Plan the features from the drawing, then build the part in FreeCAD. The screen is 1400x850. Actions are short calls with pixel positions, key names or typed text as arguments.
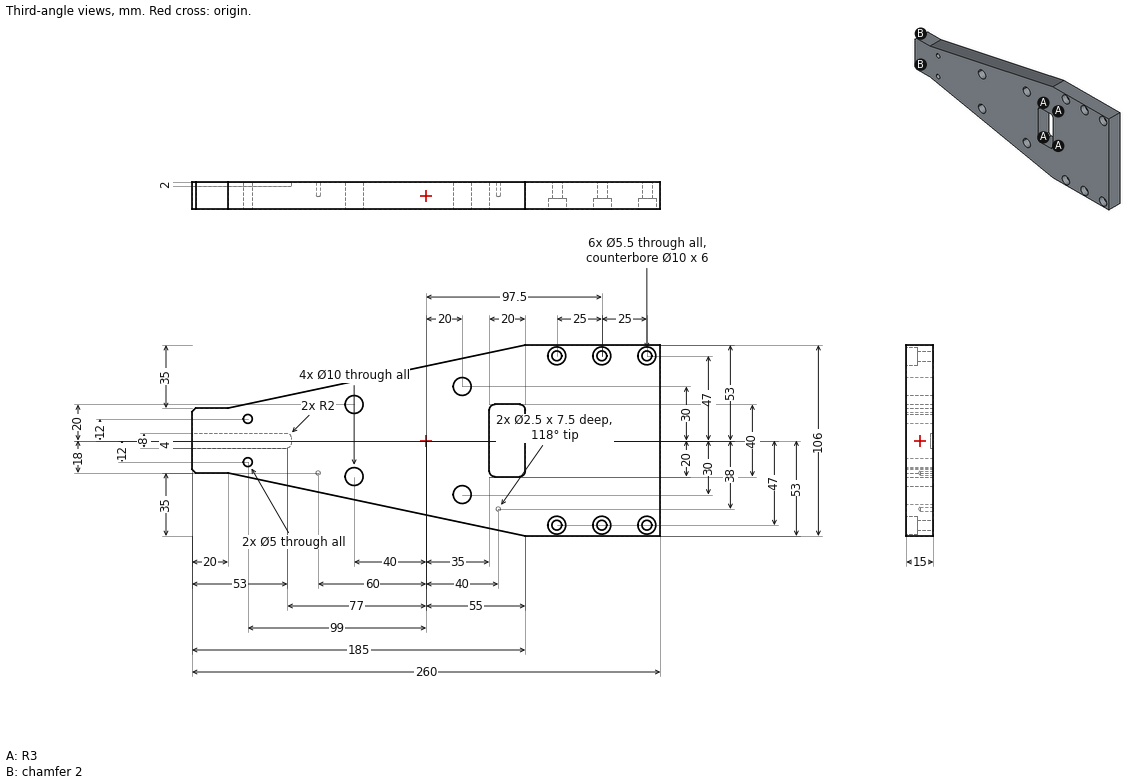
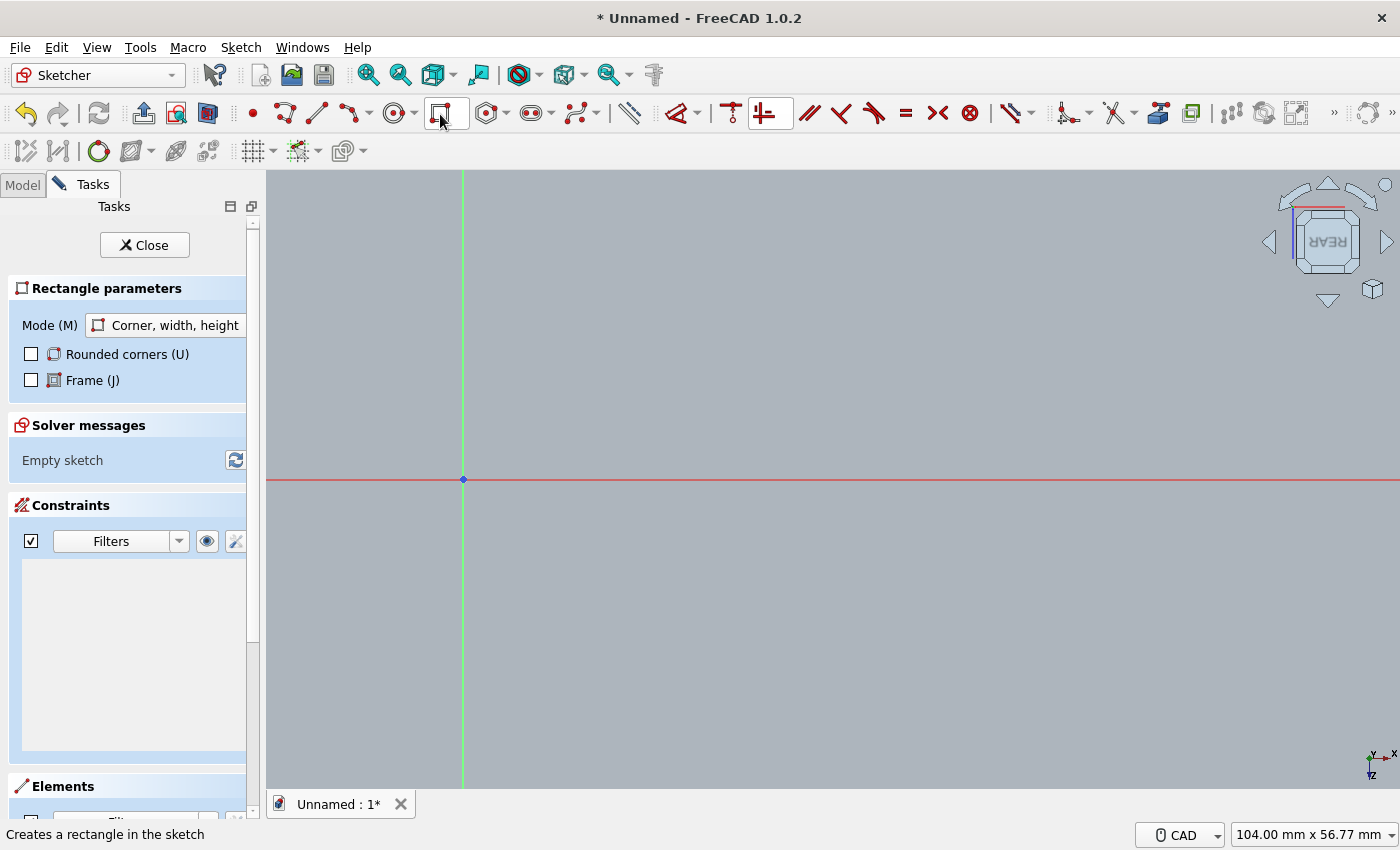
click(845, 261)
click(1063, 698)
key(Escape)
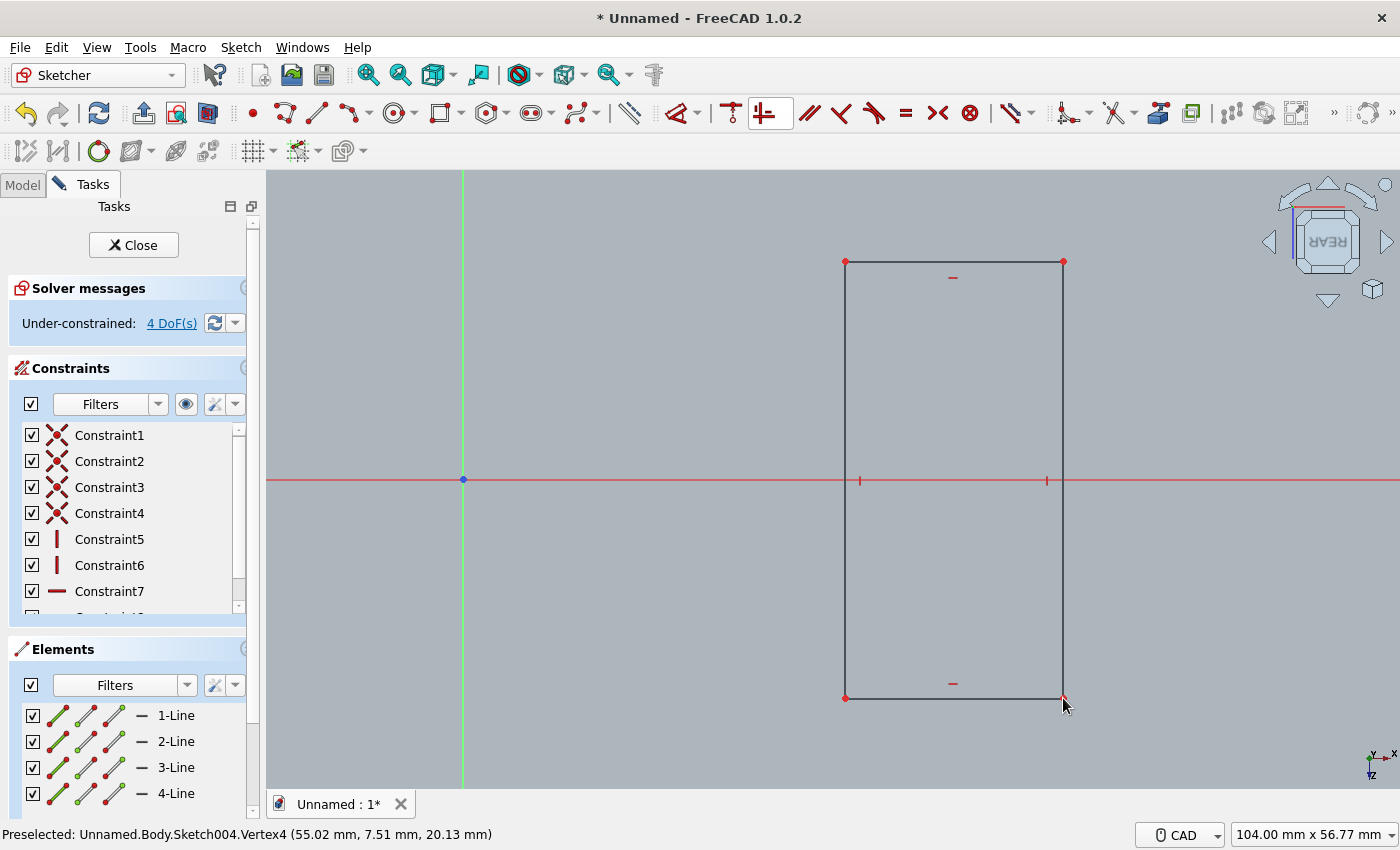
click(676, 114)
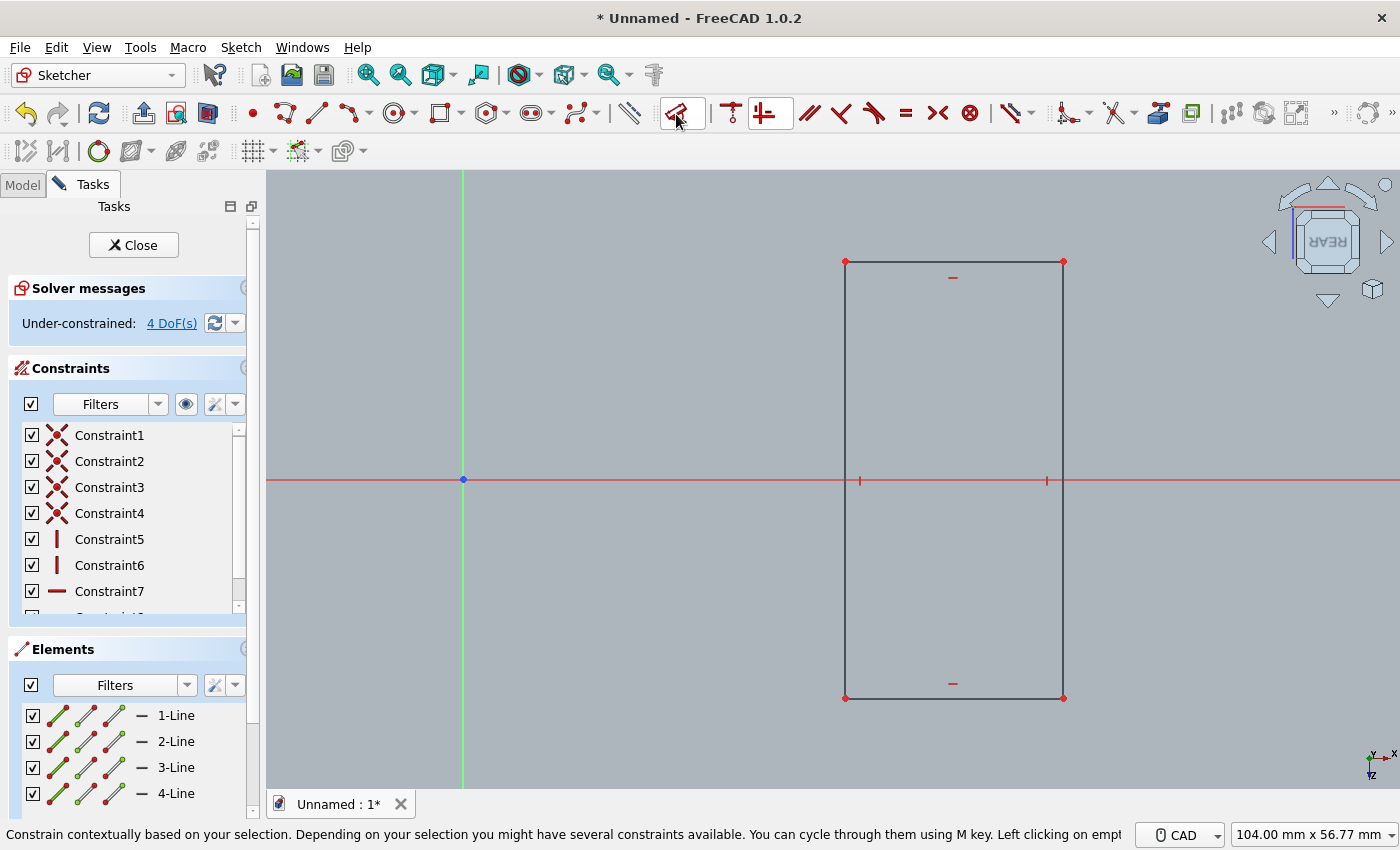
click(845, 393)
click(879, 380)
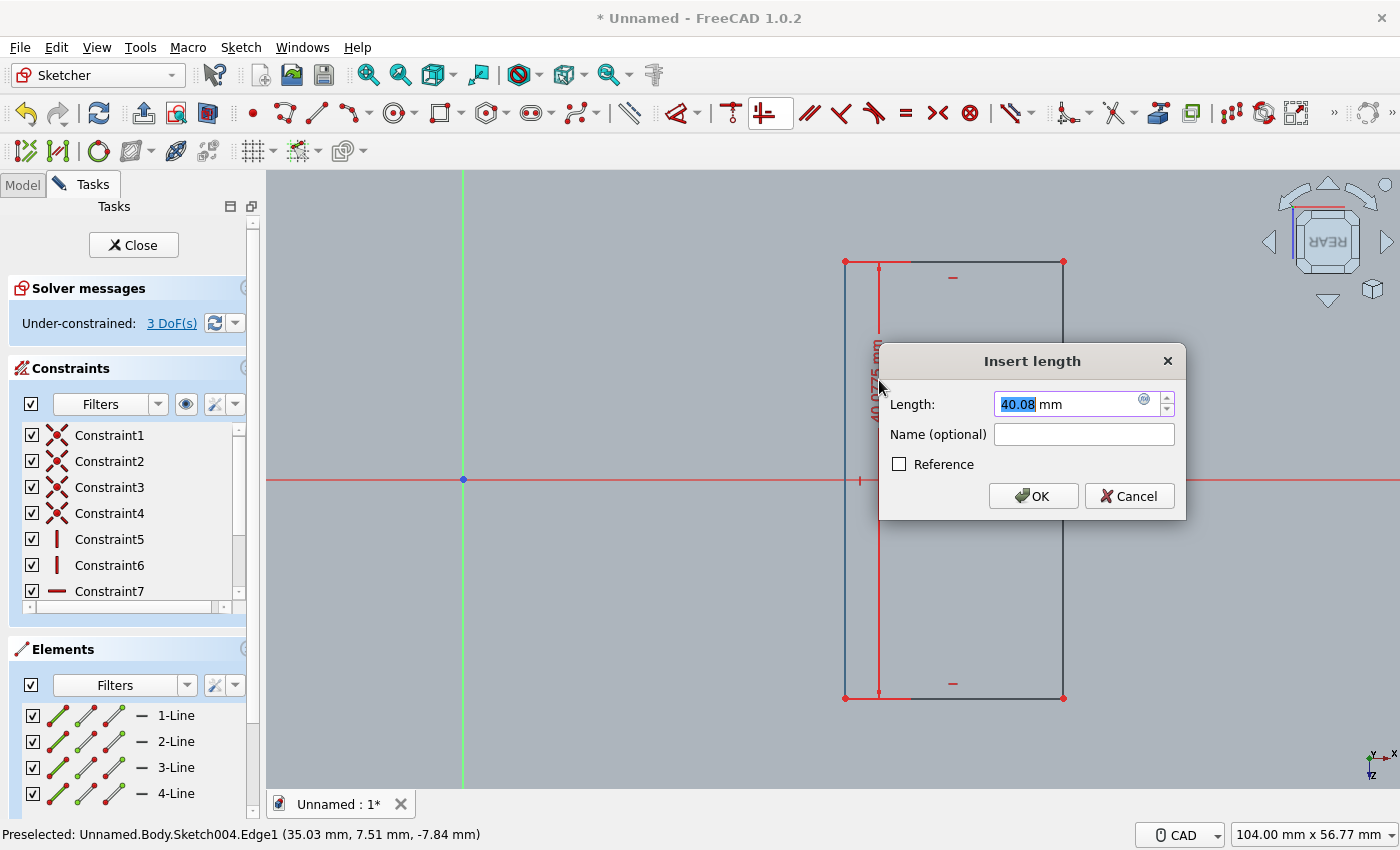
text(40)
key(Return)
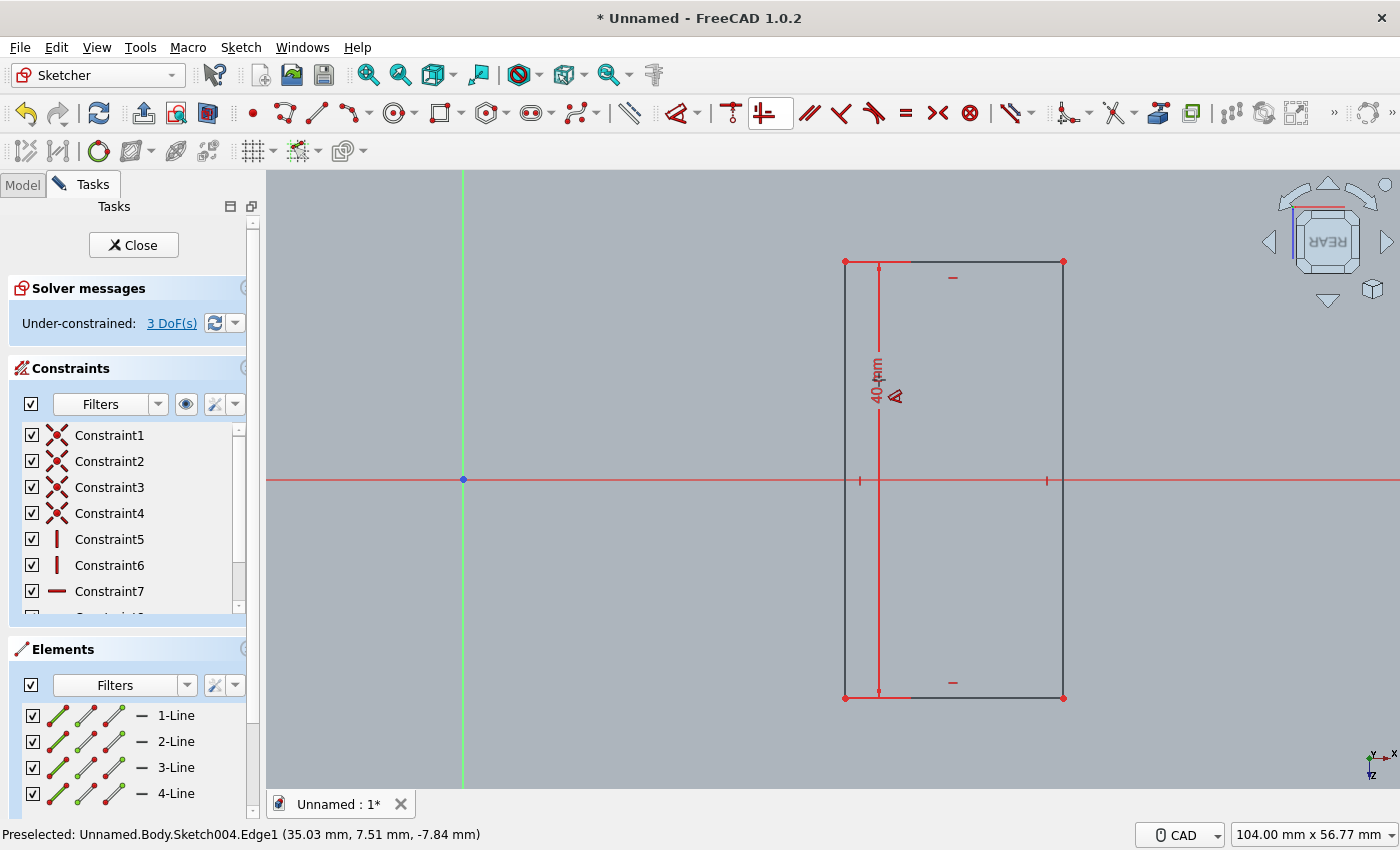
click(910, 698)
click(954, 732)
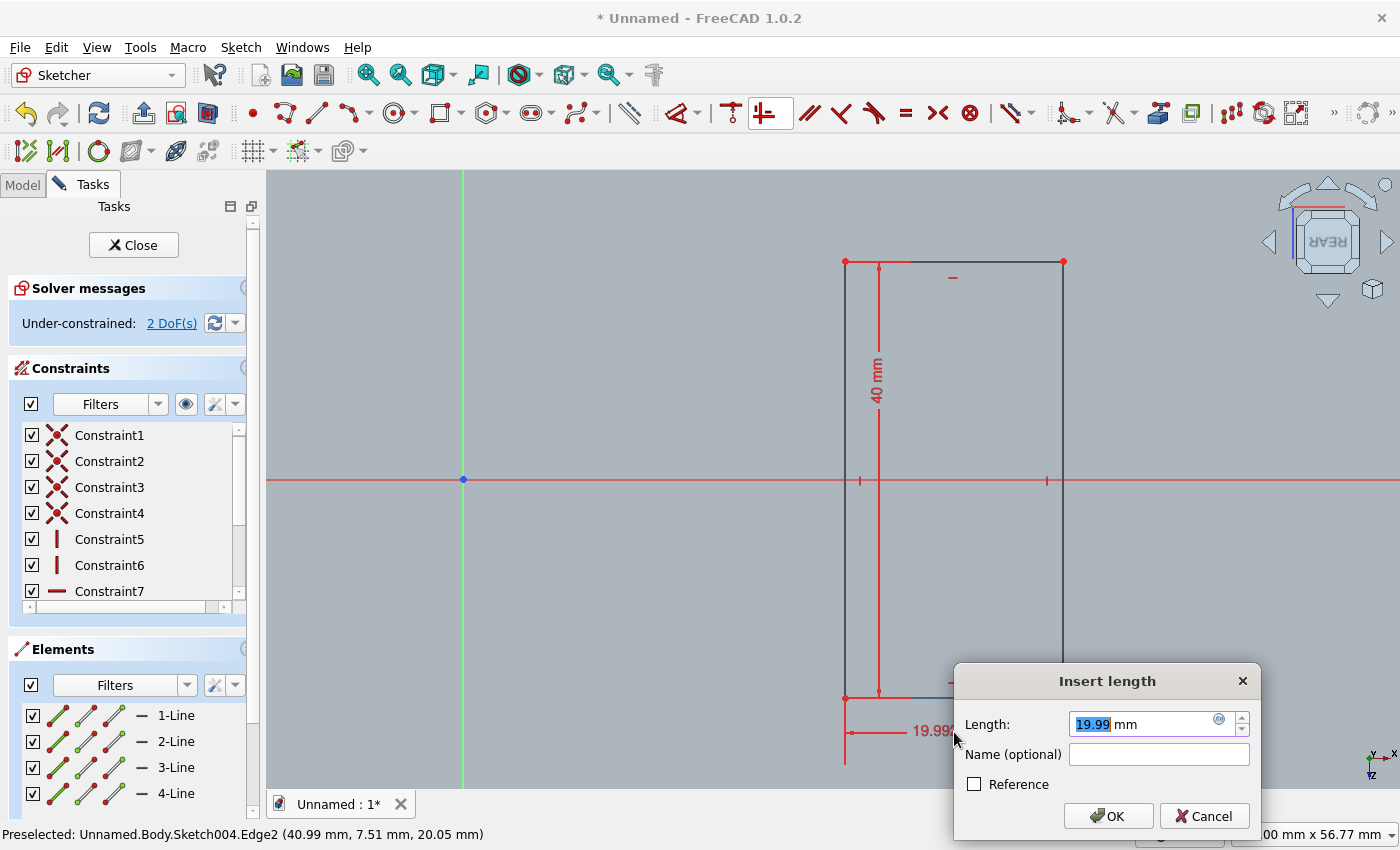
text(20)
key(Return)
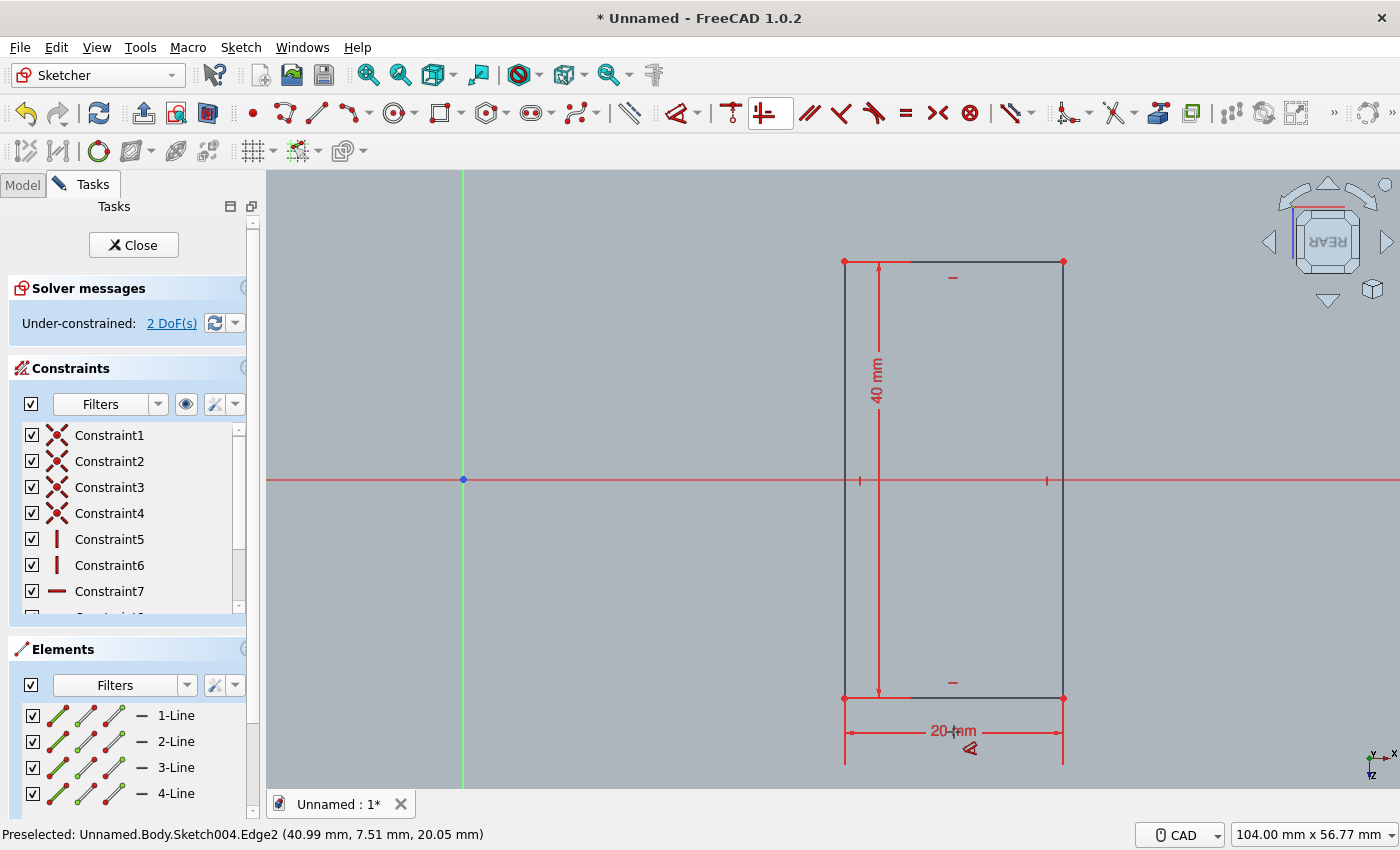
click(845, 262)
click(654, 228)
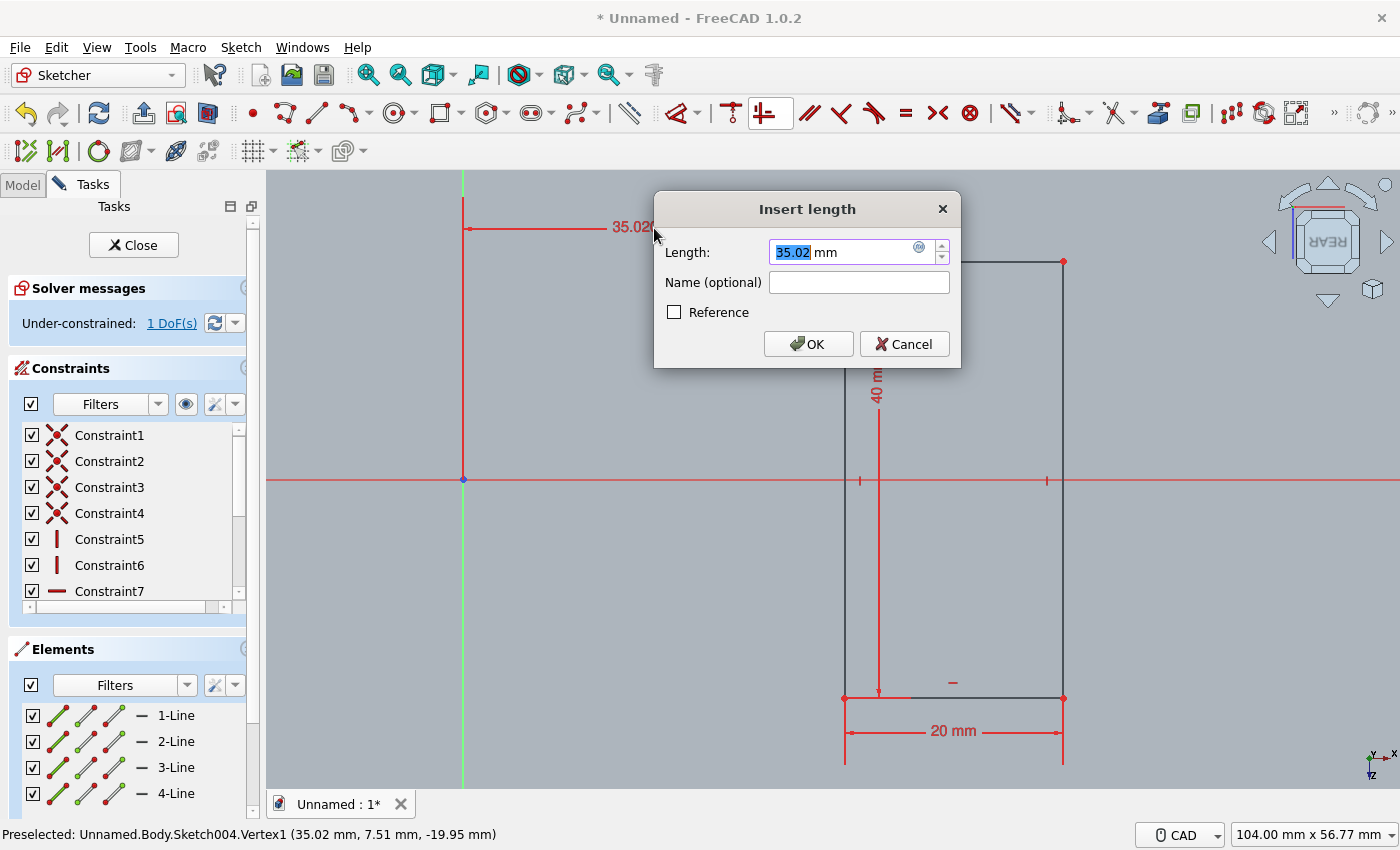
text(35)
key(Return)